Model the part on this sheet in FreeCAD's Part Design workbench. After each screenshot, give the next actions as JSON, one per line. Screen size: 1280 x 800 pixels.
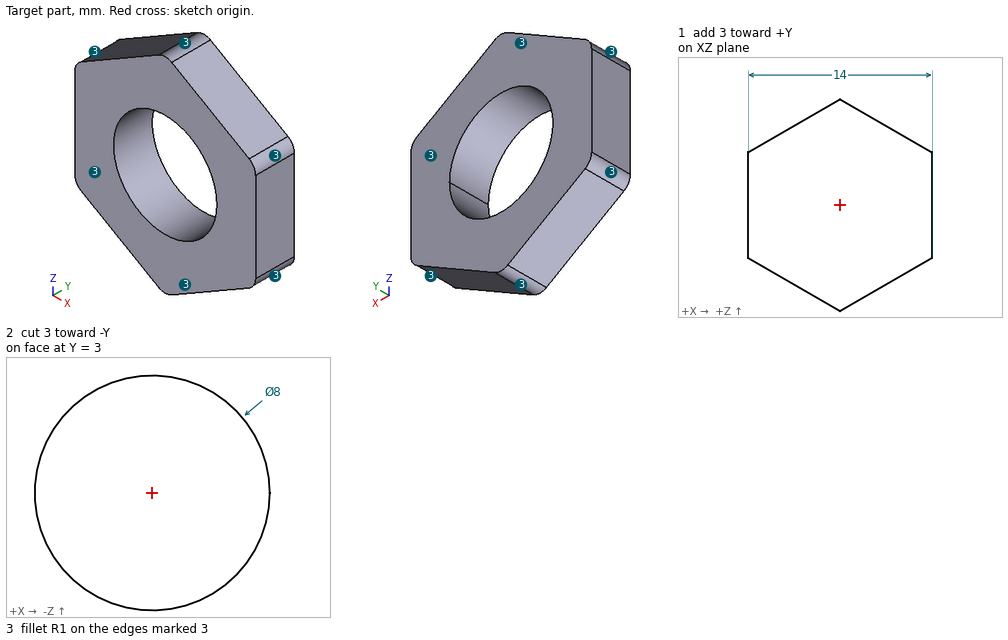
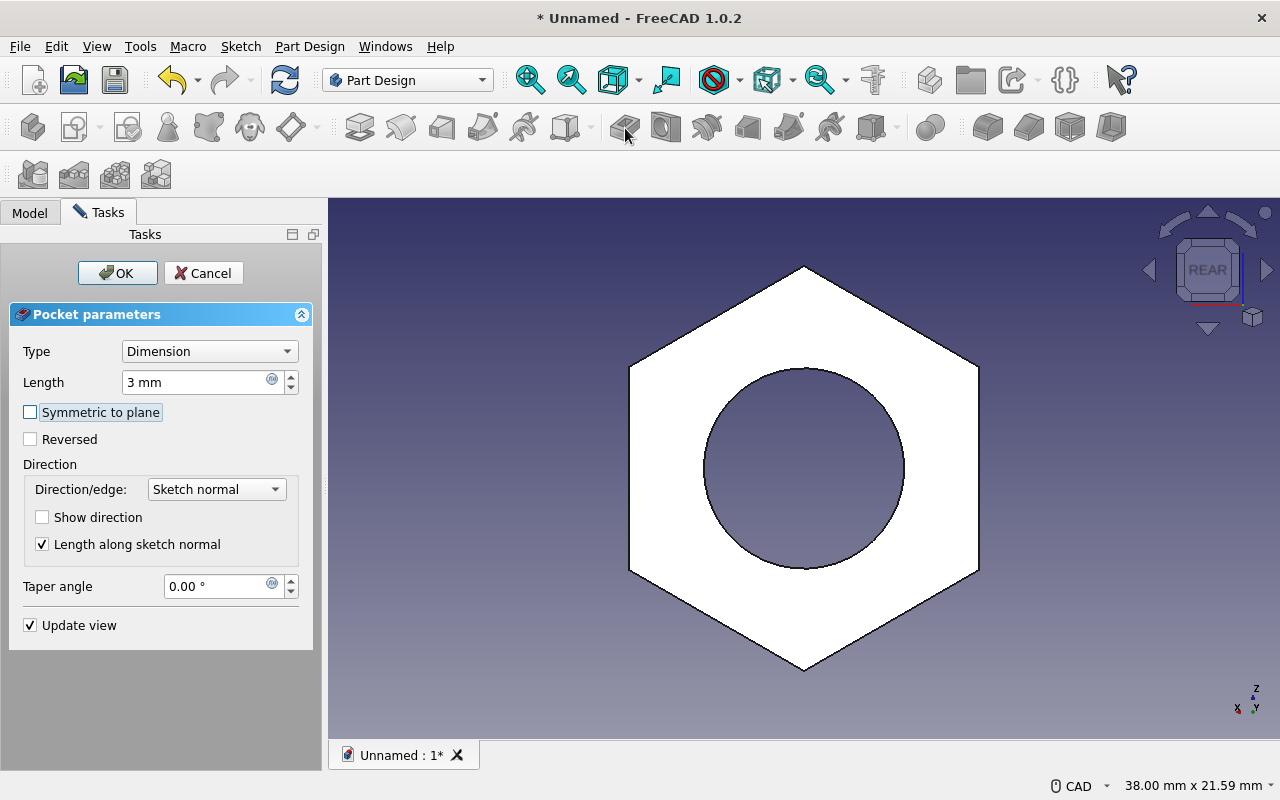
{"action": "left_click", "coordinate": [118, 273]}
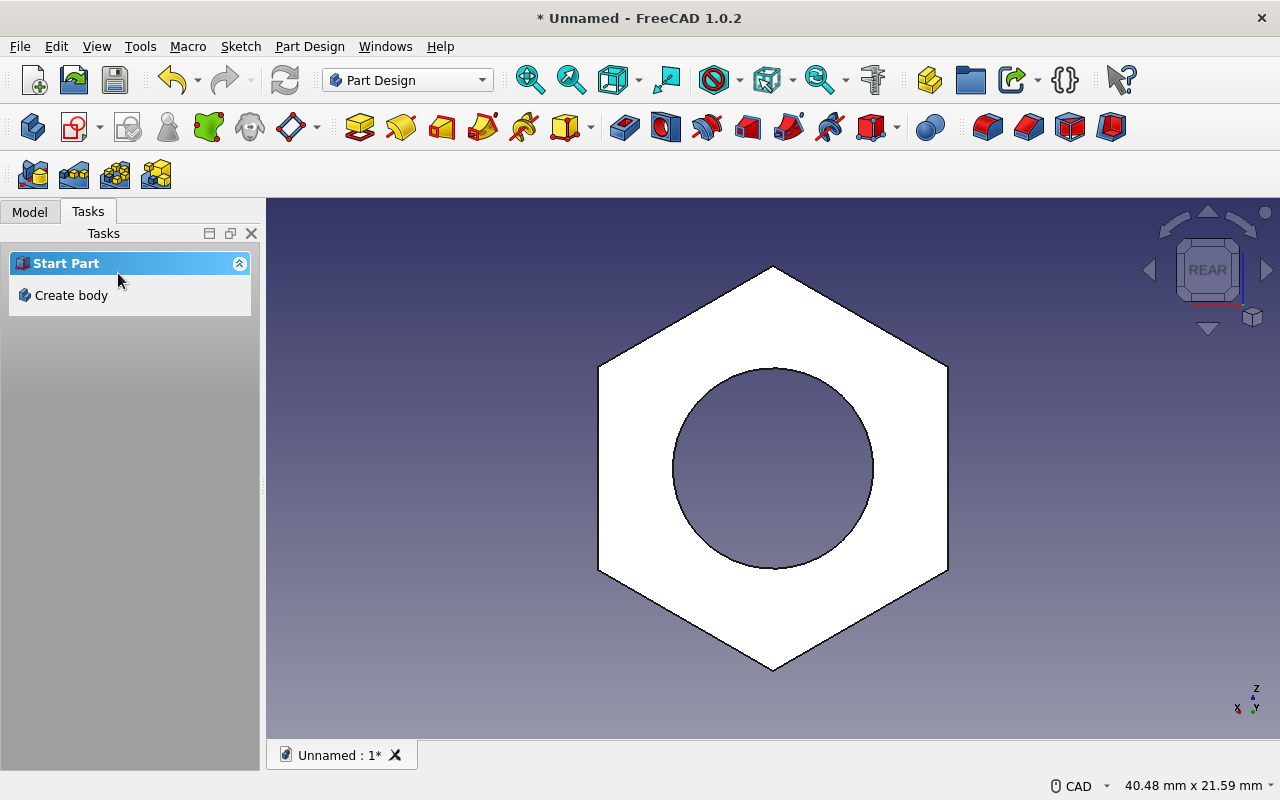
{"action": "key", "text": "0"}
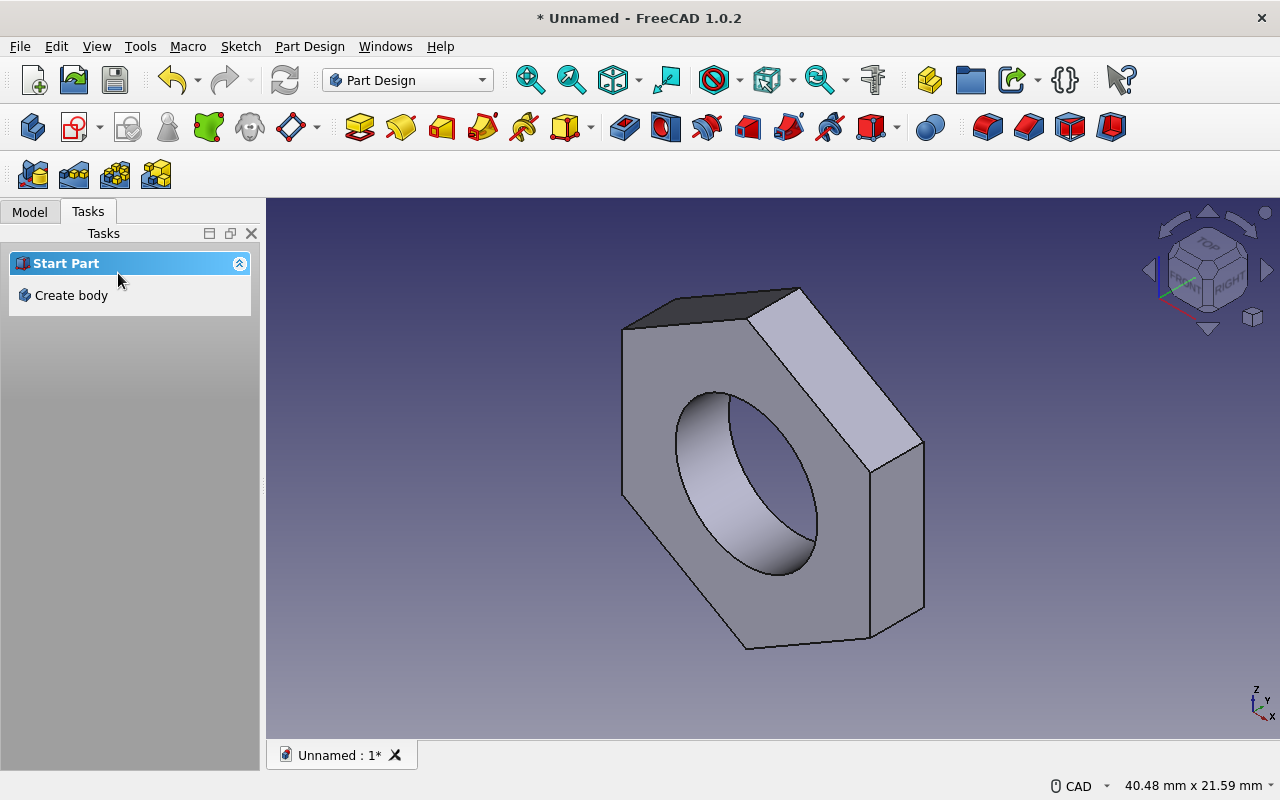
{"action": "left_click", "coordinate": [897, 456]}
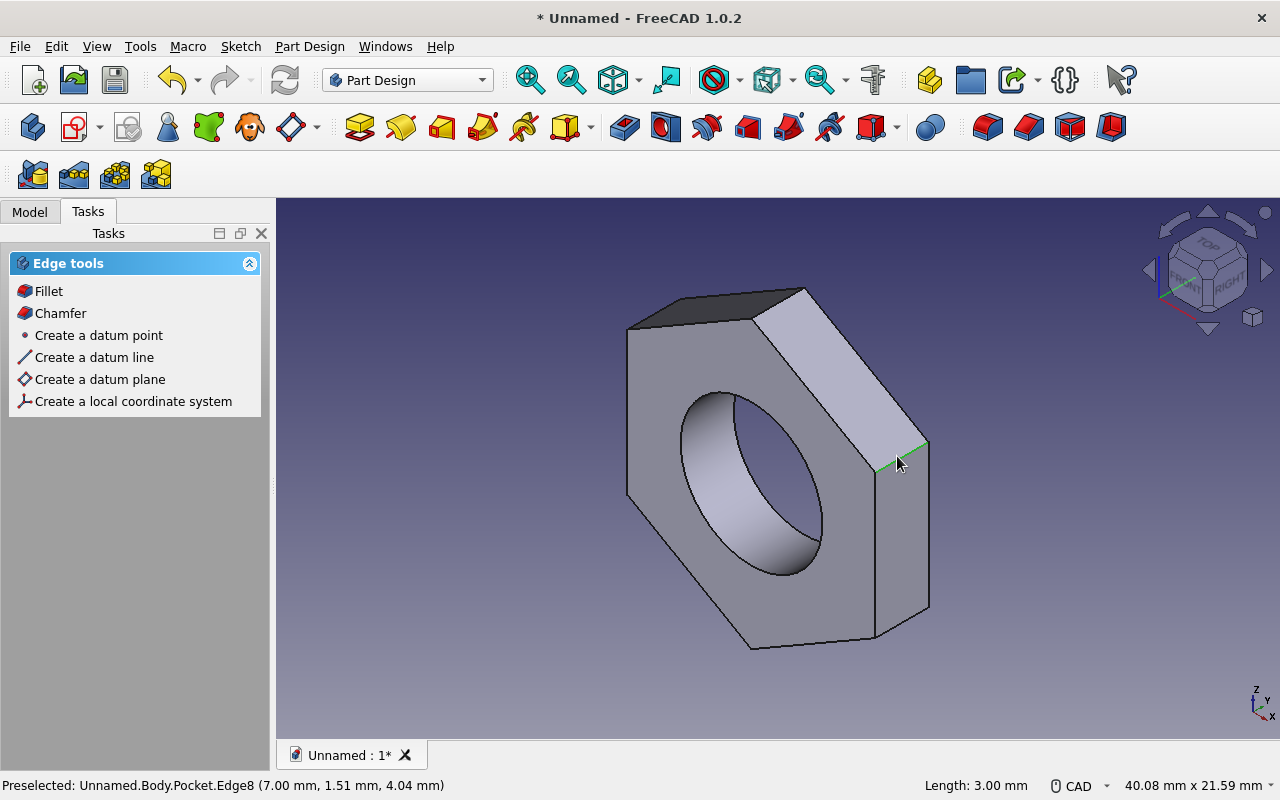
{"action": "key", "text": "2"}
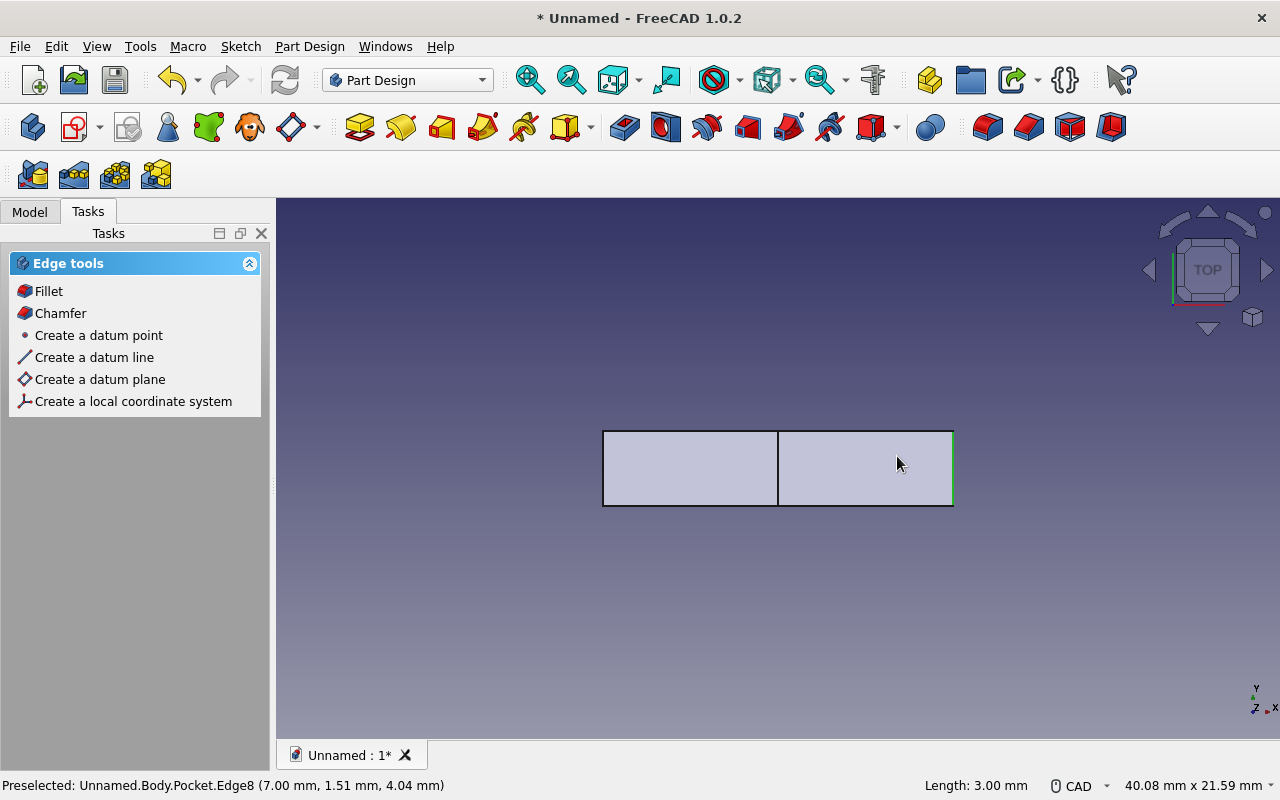
{"action": "key", "text": "v f"}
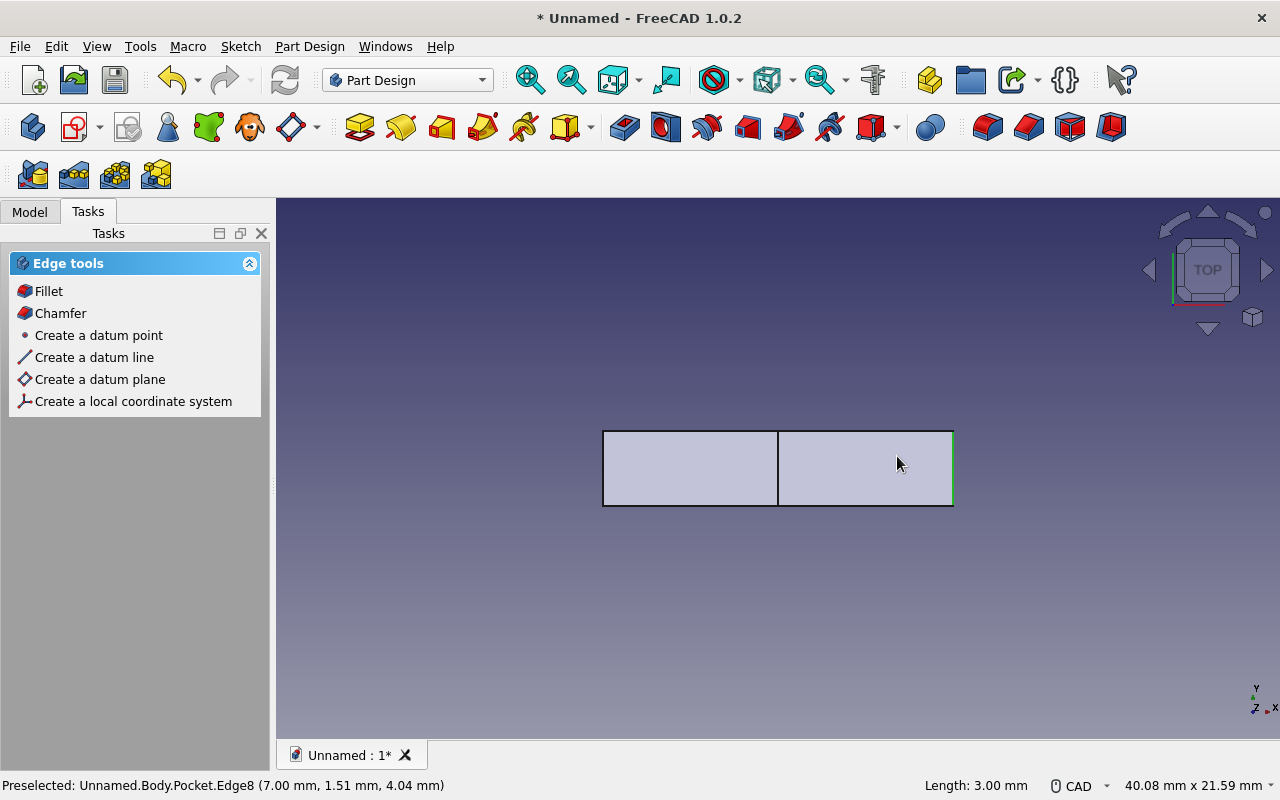
{"action": "left_click", "coordinate": [778, 467], "text": "ctrl"}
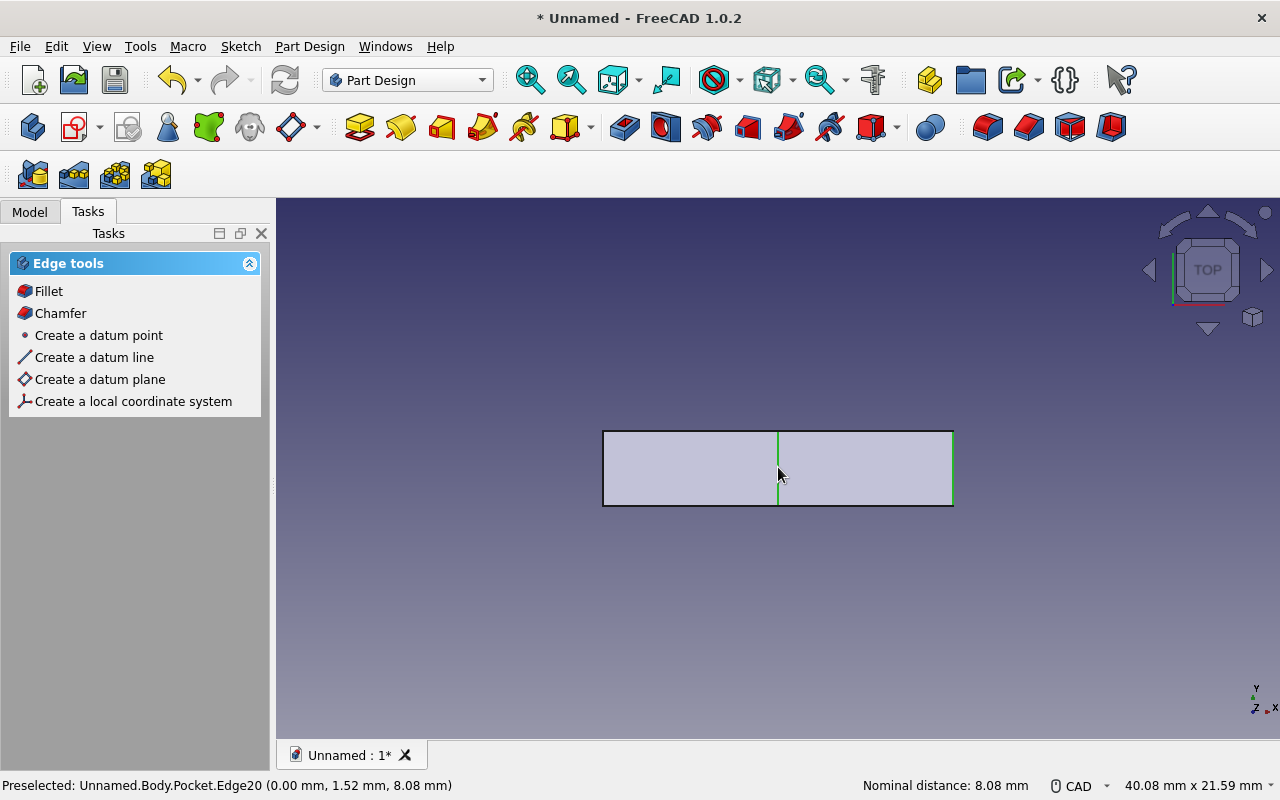
{"action": "key", "text": "1"}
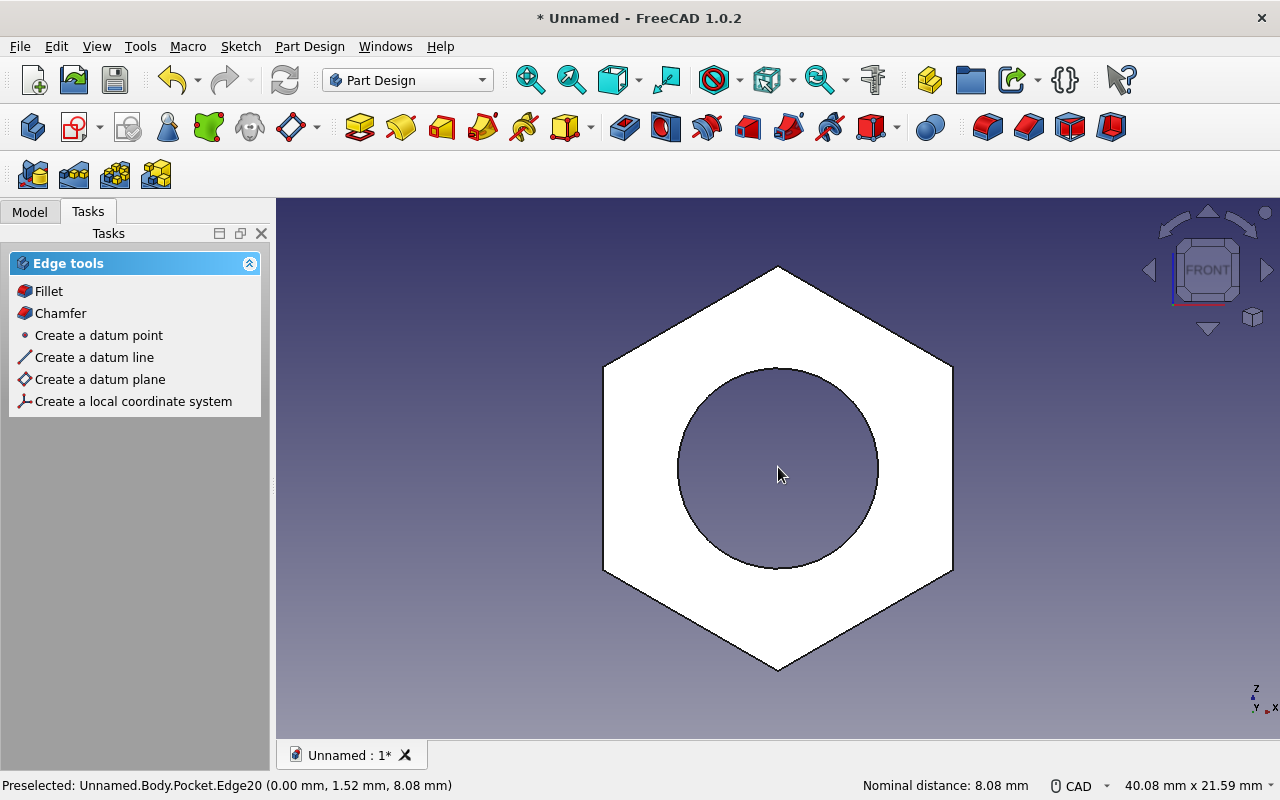
{"action": "key", "text": "3"}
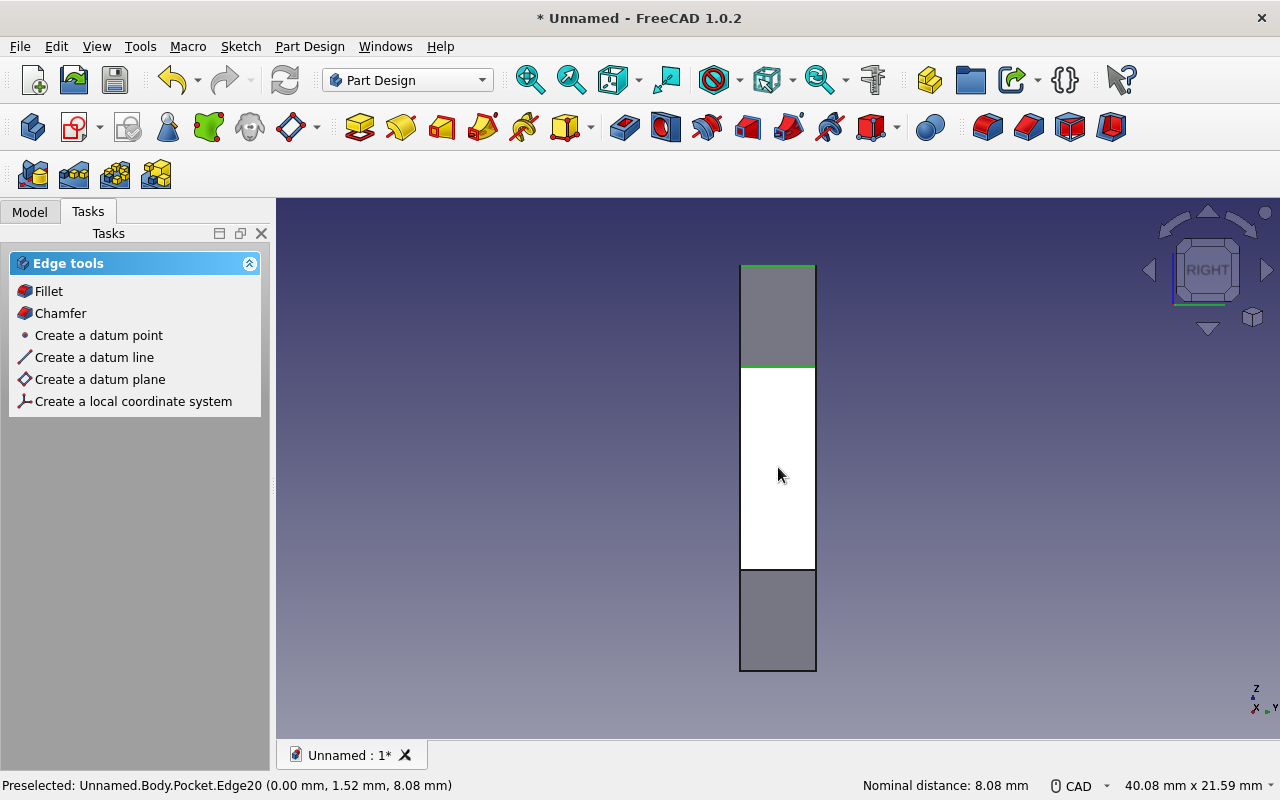
{"action": "left_click", "coordinate": [778, 569], "text": "ctrl"}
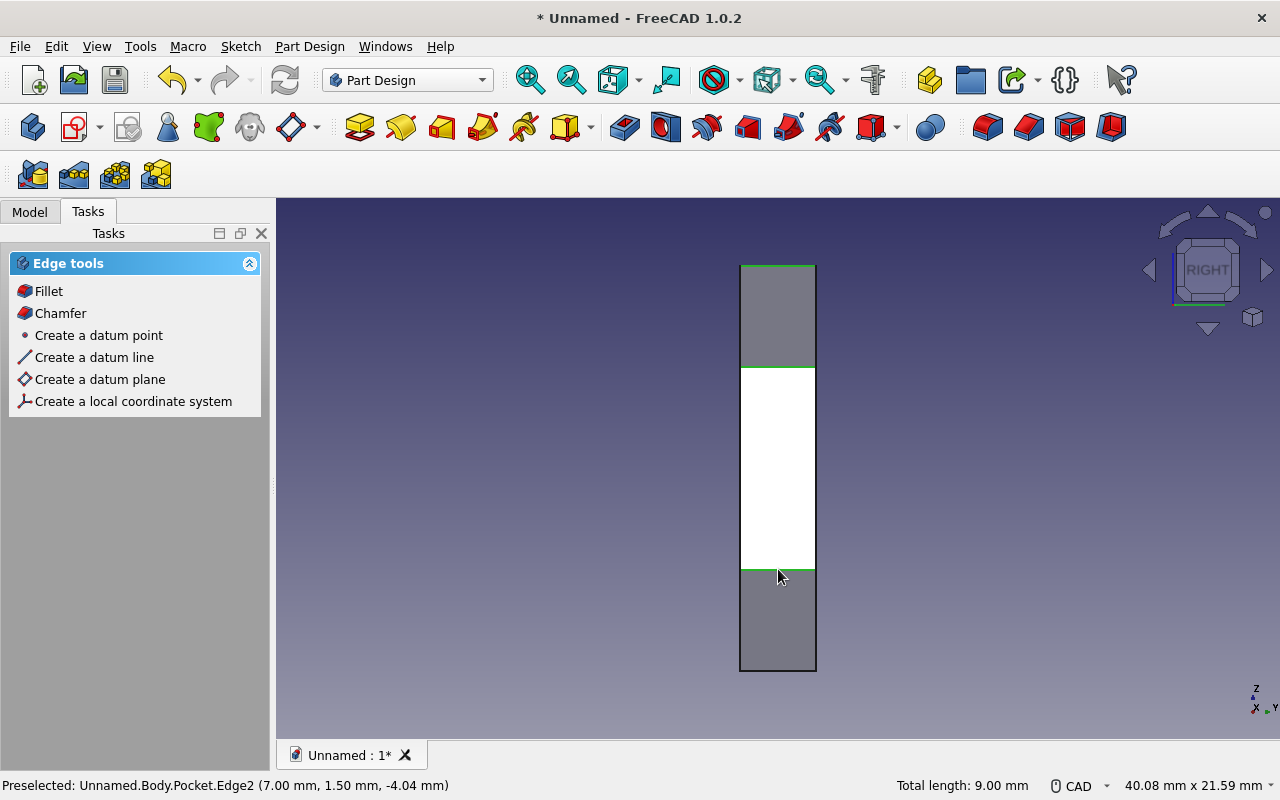
{"action": "key", "text": "5"}